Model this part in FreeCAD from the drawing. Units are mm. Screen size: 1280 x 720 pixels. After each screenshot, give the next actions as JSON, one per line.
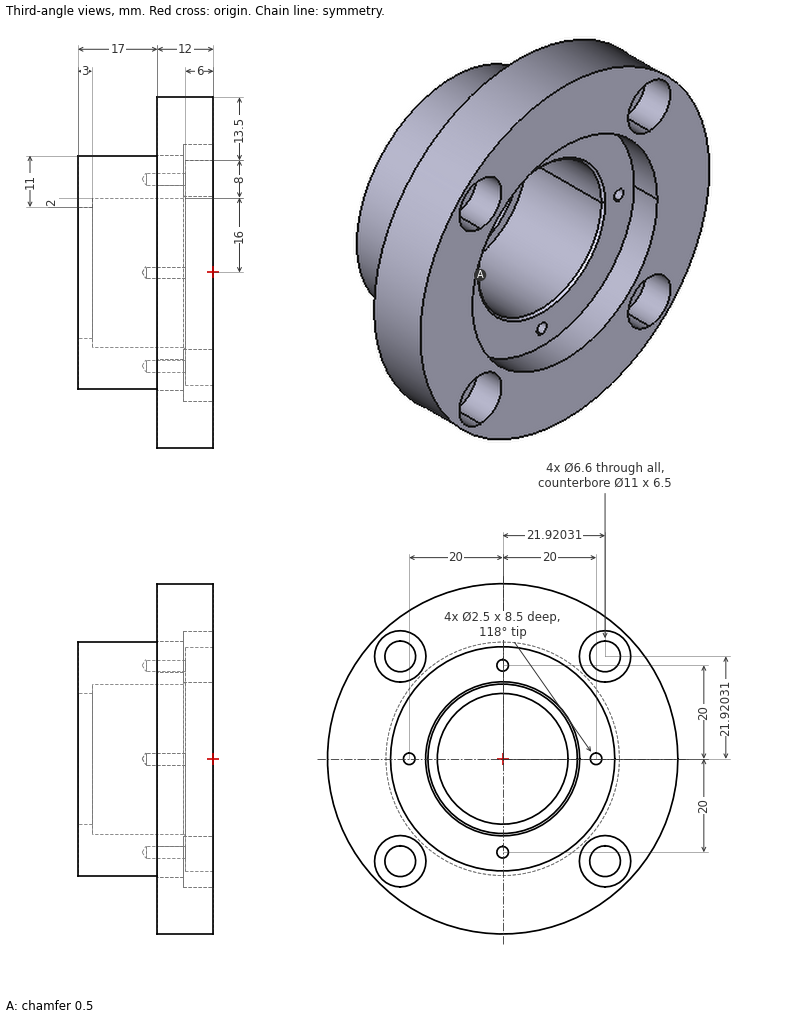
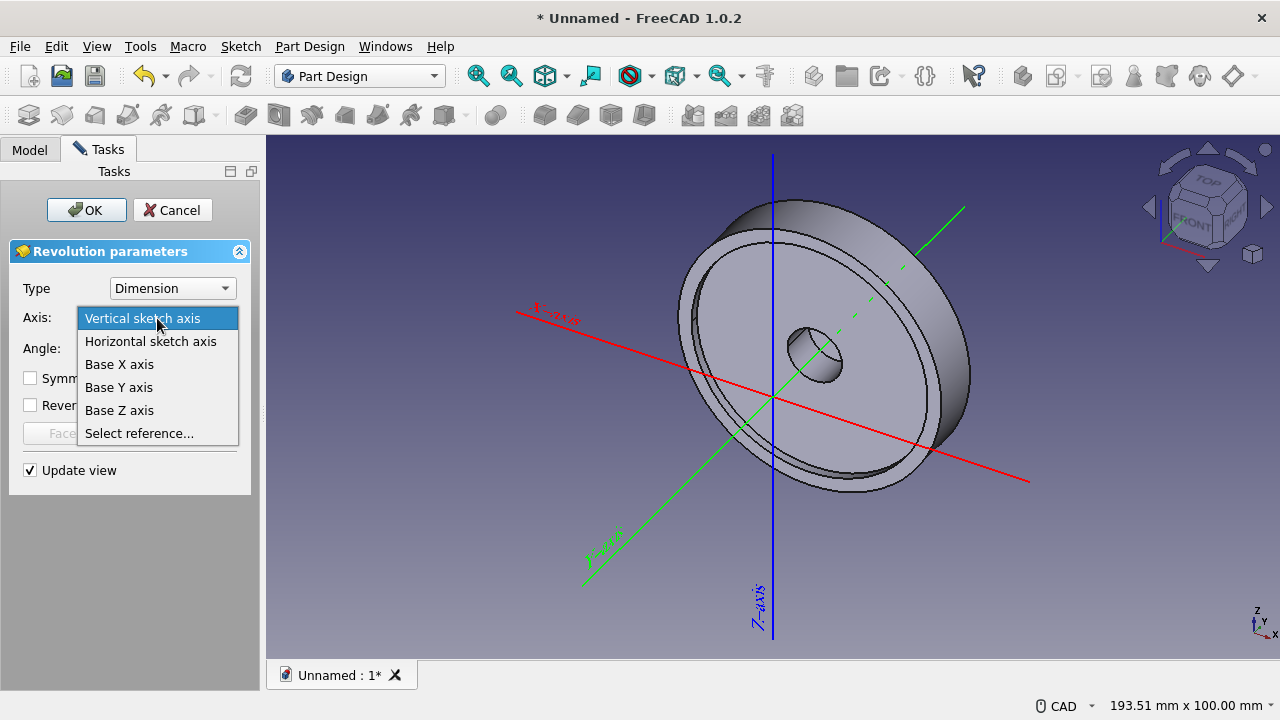
{"action": "left_click", "coordinate": [156, 342]}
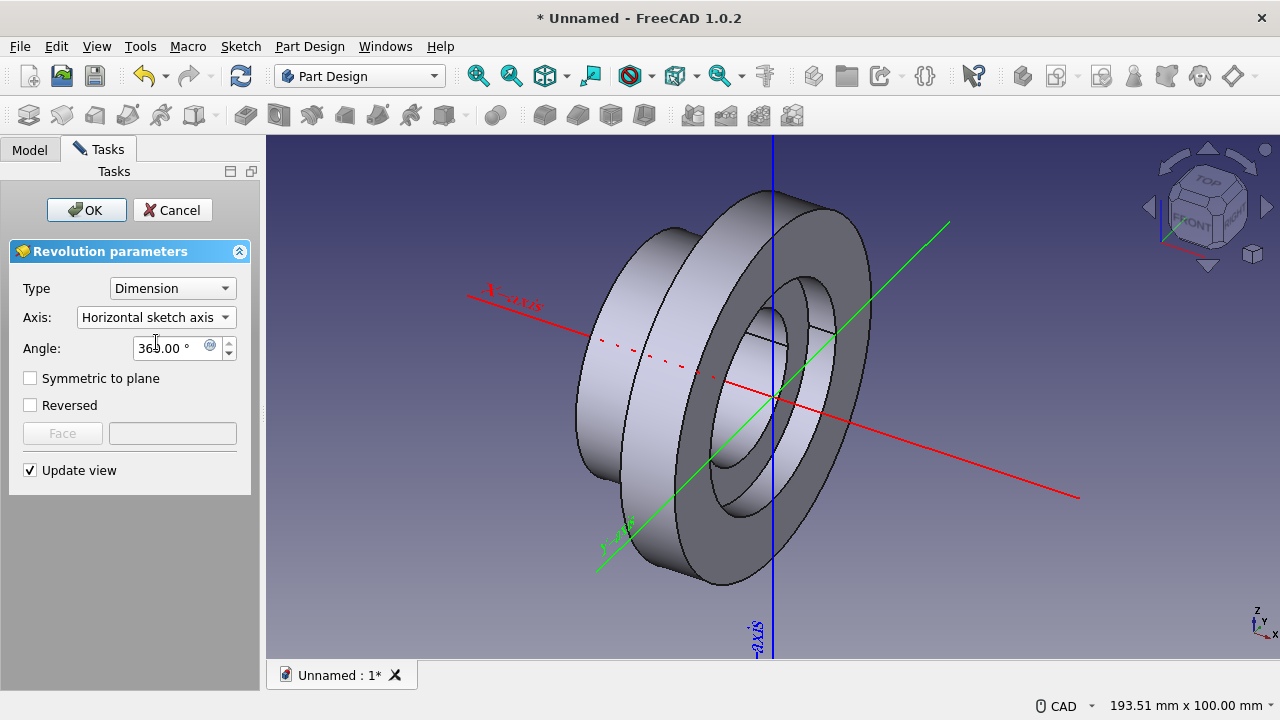
{"action": "left_click", "coordinate": [87, 210]}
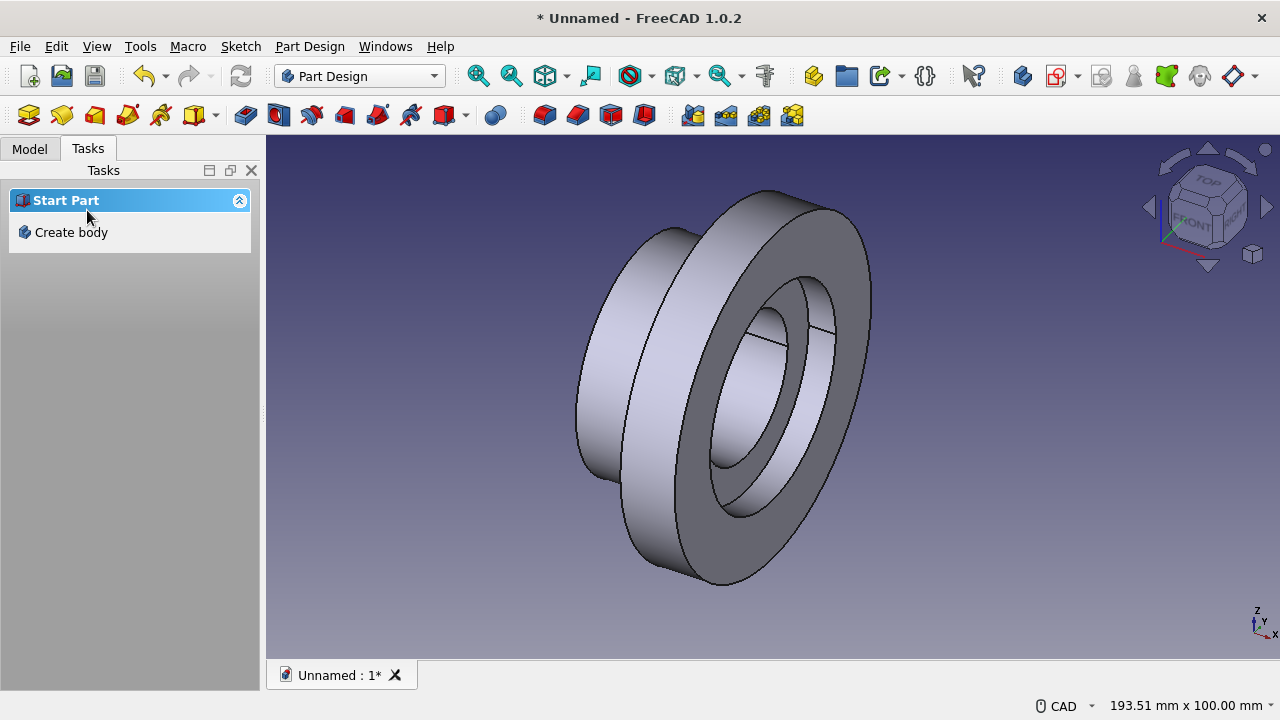
{"action": "key", "text": "v f"}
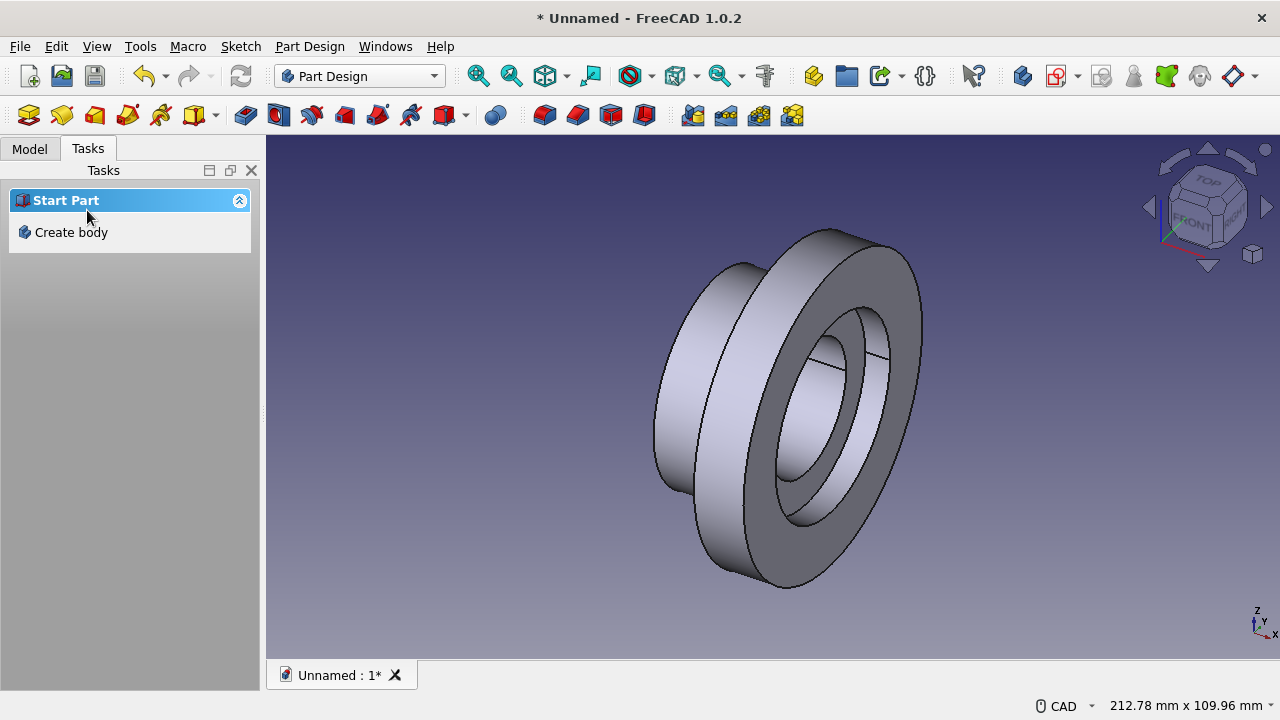
{"action": "left_click", "coordinate": [782, 383]}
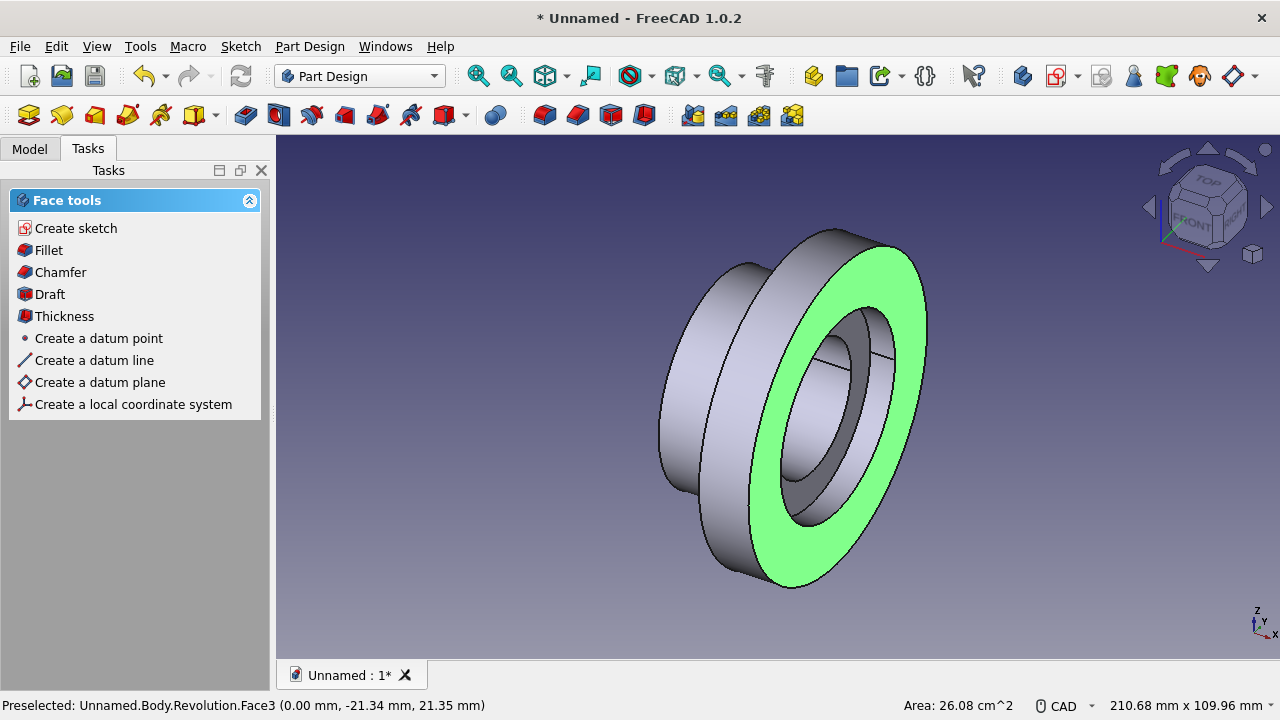
{"action": "left_click", "coordinate": [1056, 76]}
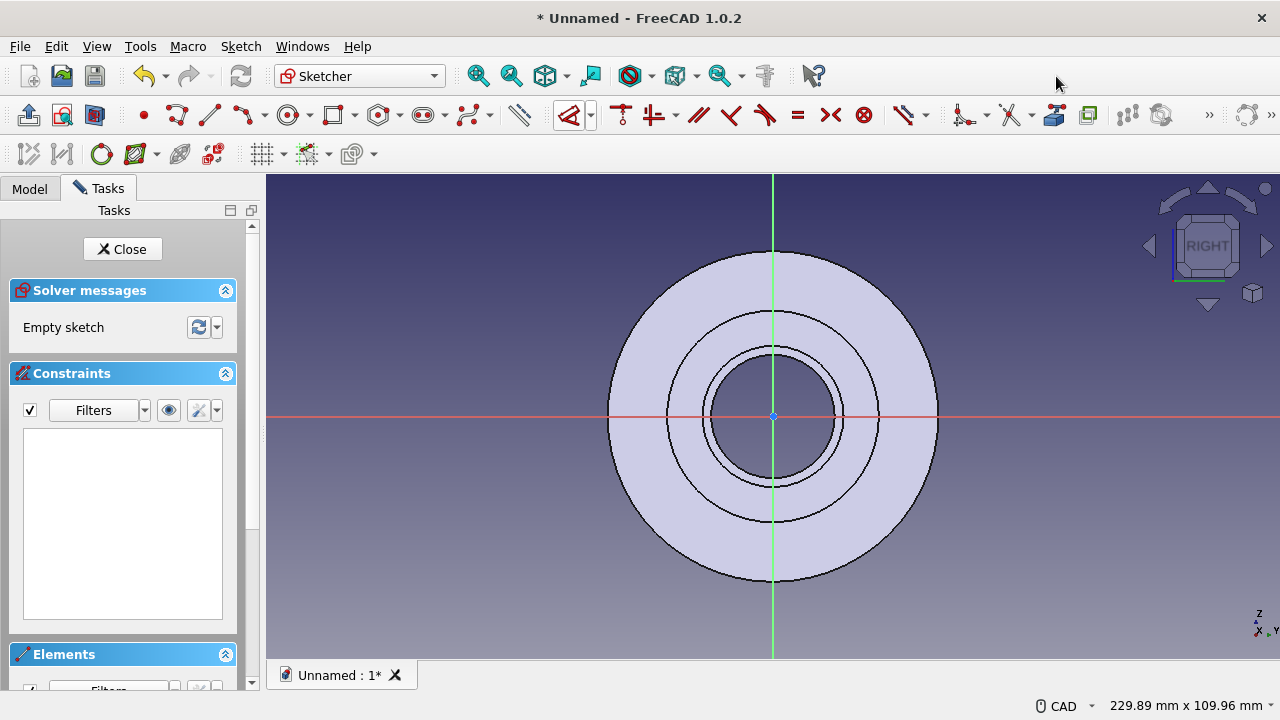
{"action": "scroll", "coordinate": [912, 416], "scroll_direction": "up", "scroll_amount": 2}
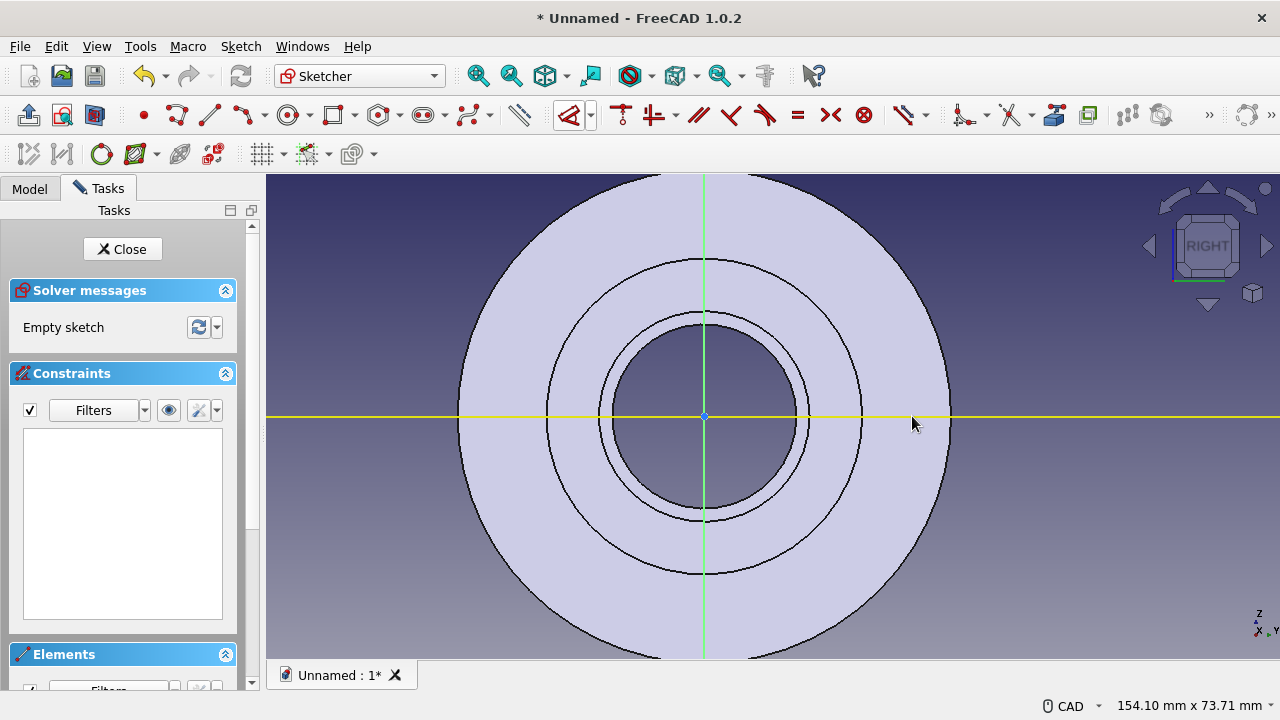
{"action": "key", "text": "g c"}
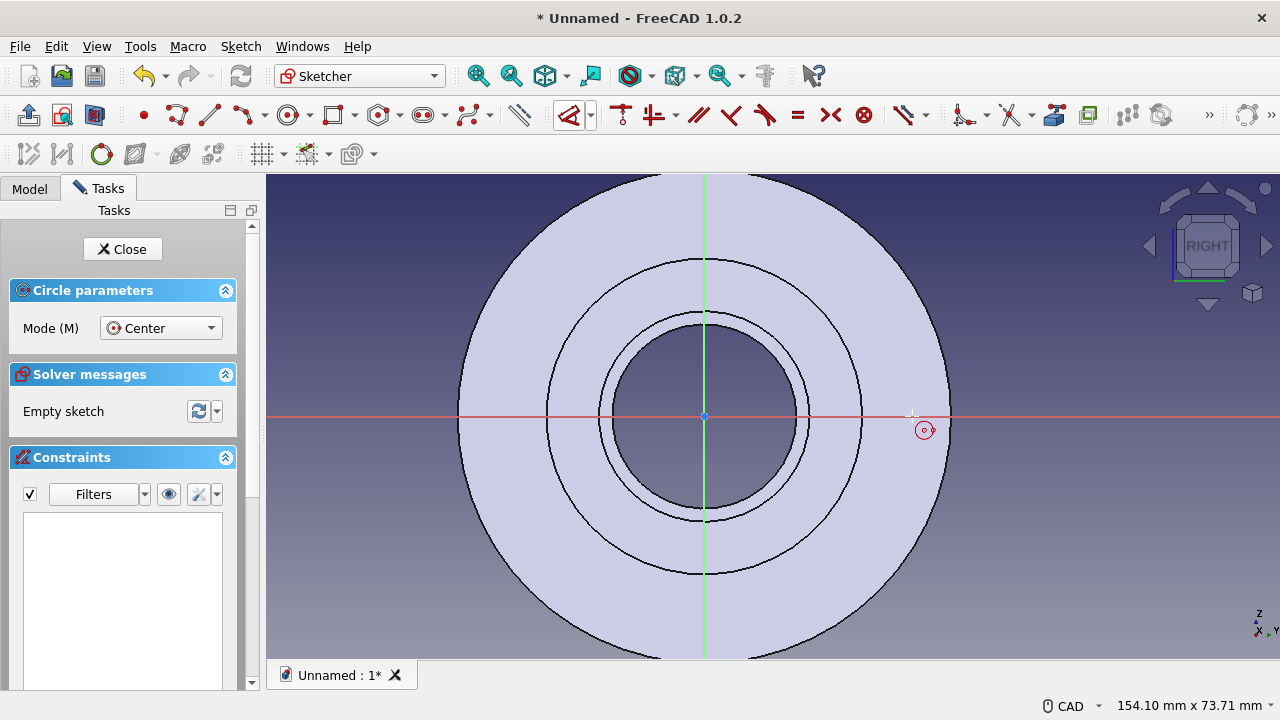
{"action": "left_click", "coordinate": [849, 272]}
{"action": "left_click", "coordinate": [864, 257]}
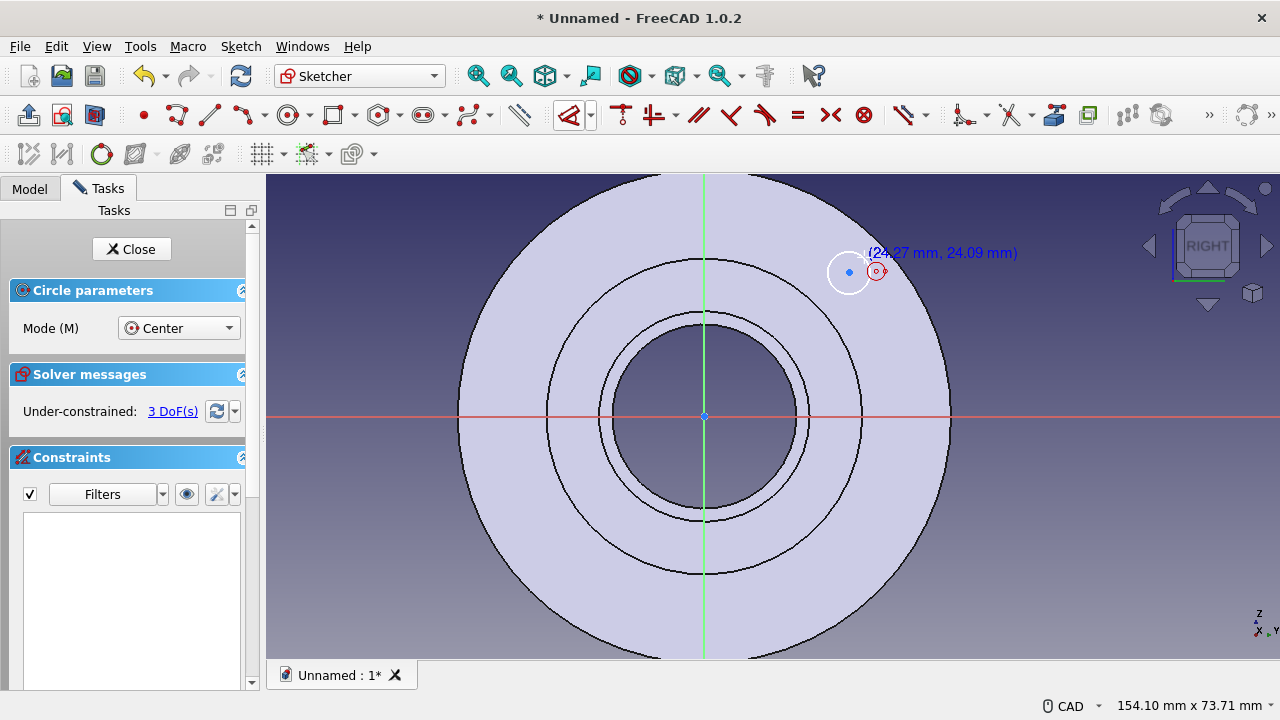
{"action": "left_click", "coordinate": [849, 561]}
{"action": "left_click", "coordinate": [864, 545]}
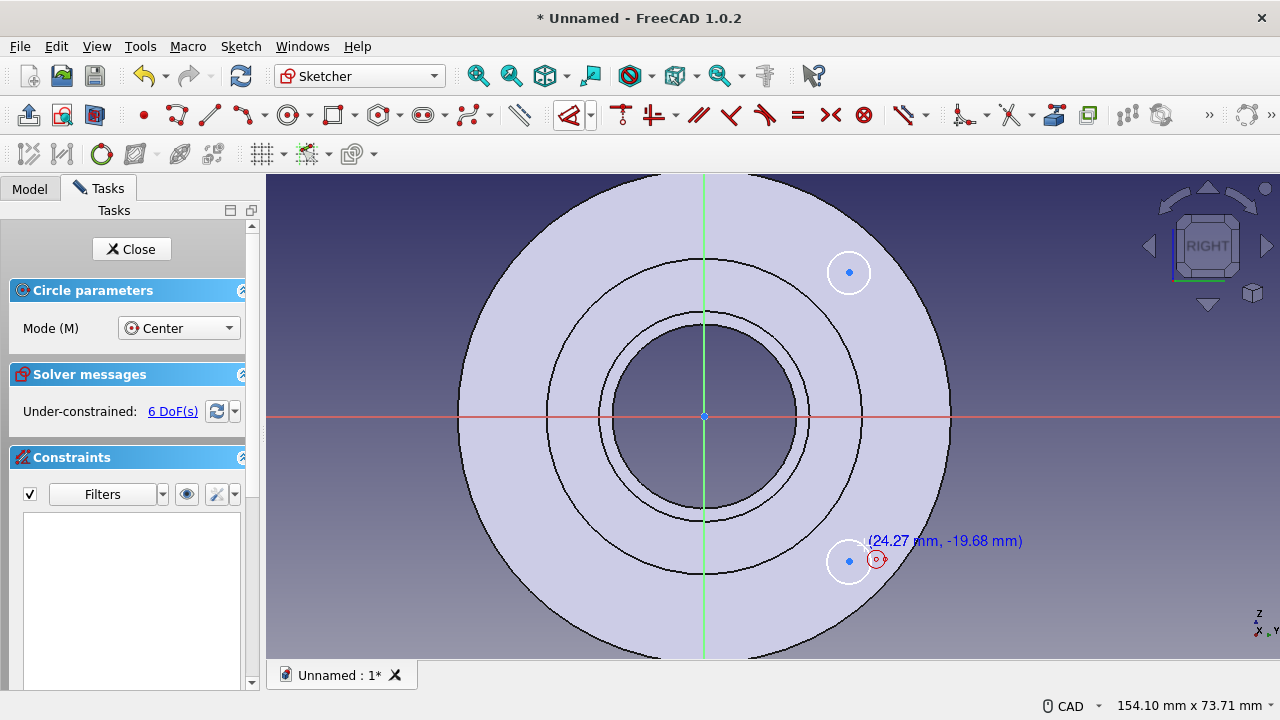
{"action": "left_click", "coordinate": [560, 561]}
{"action": "left_click", "coordinate": [575, 545]}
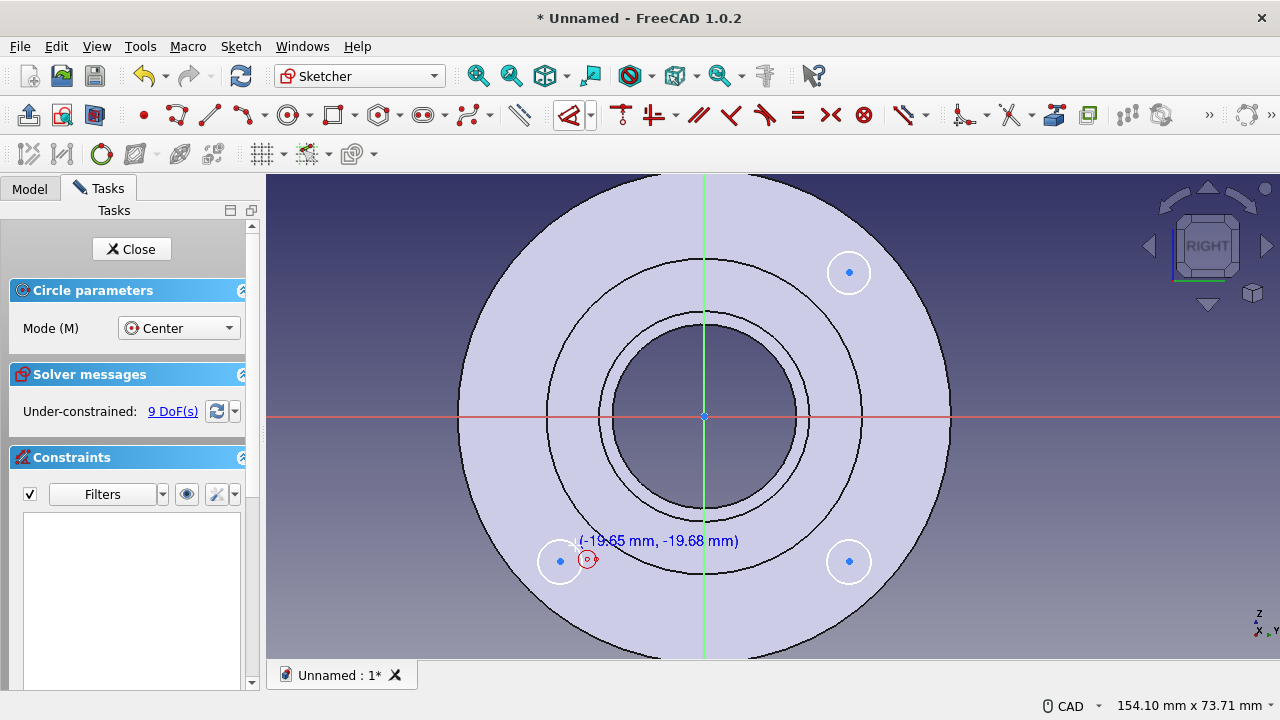
{"action": "left_click", "coordinate": [560, 272]}
{"action": "left_click", "coordinate": [575, 257]}
{"action": "key", "text": "Escape"}